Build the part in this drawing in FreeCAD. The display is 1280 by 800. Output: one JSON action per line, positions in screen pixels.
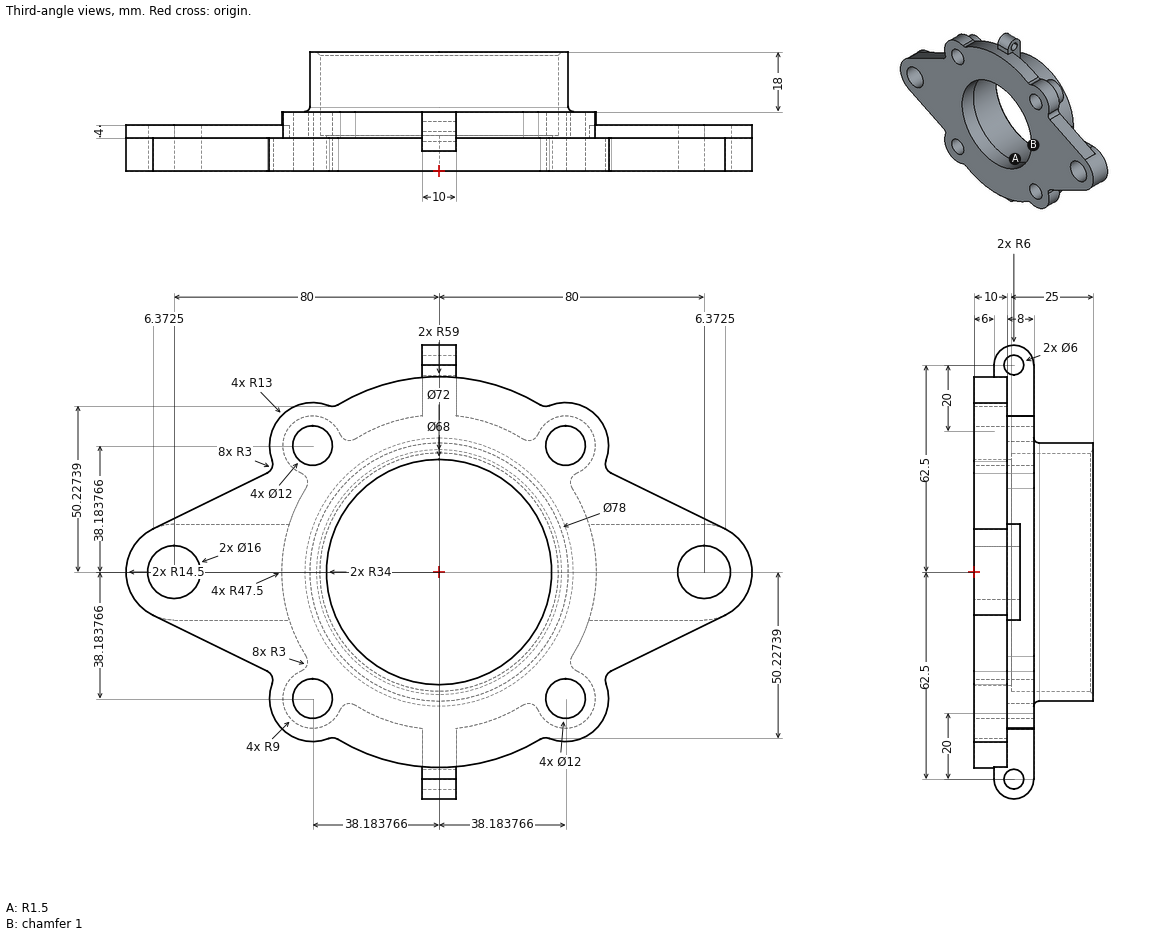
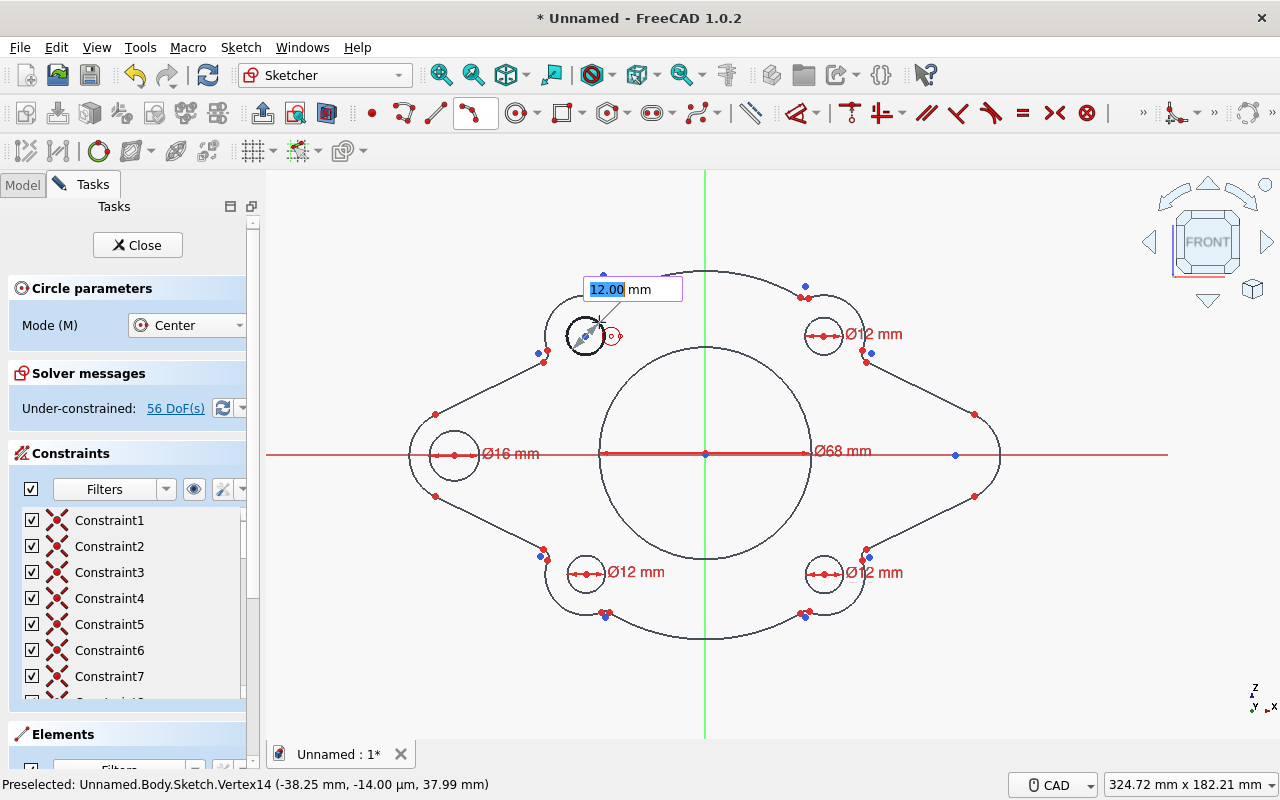
{"action": "type", "text": "12"}
{"action": "key", "text": "Return"}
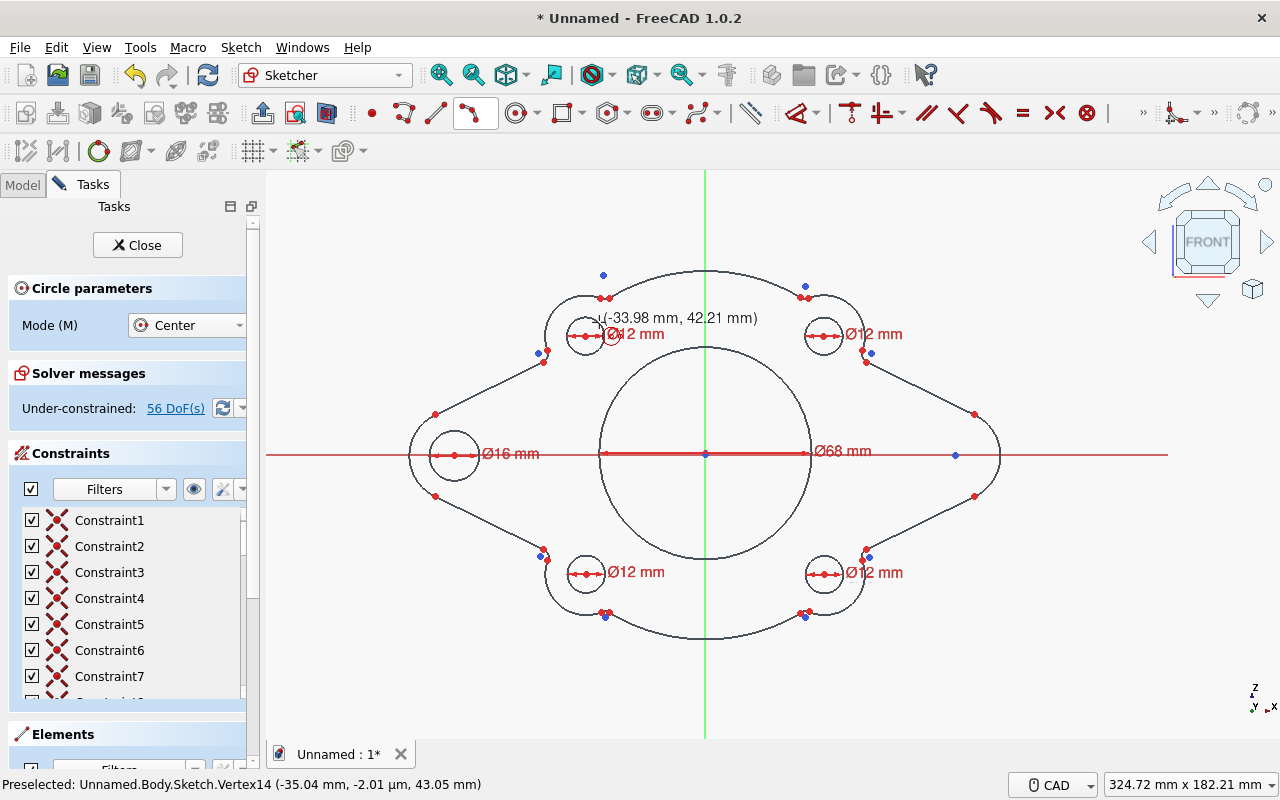
{"action": "left_click", "coordinate": [955, 455]}
{"action": "mouse_move", "coordinate": [973, 437]}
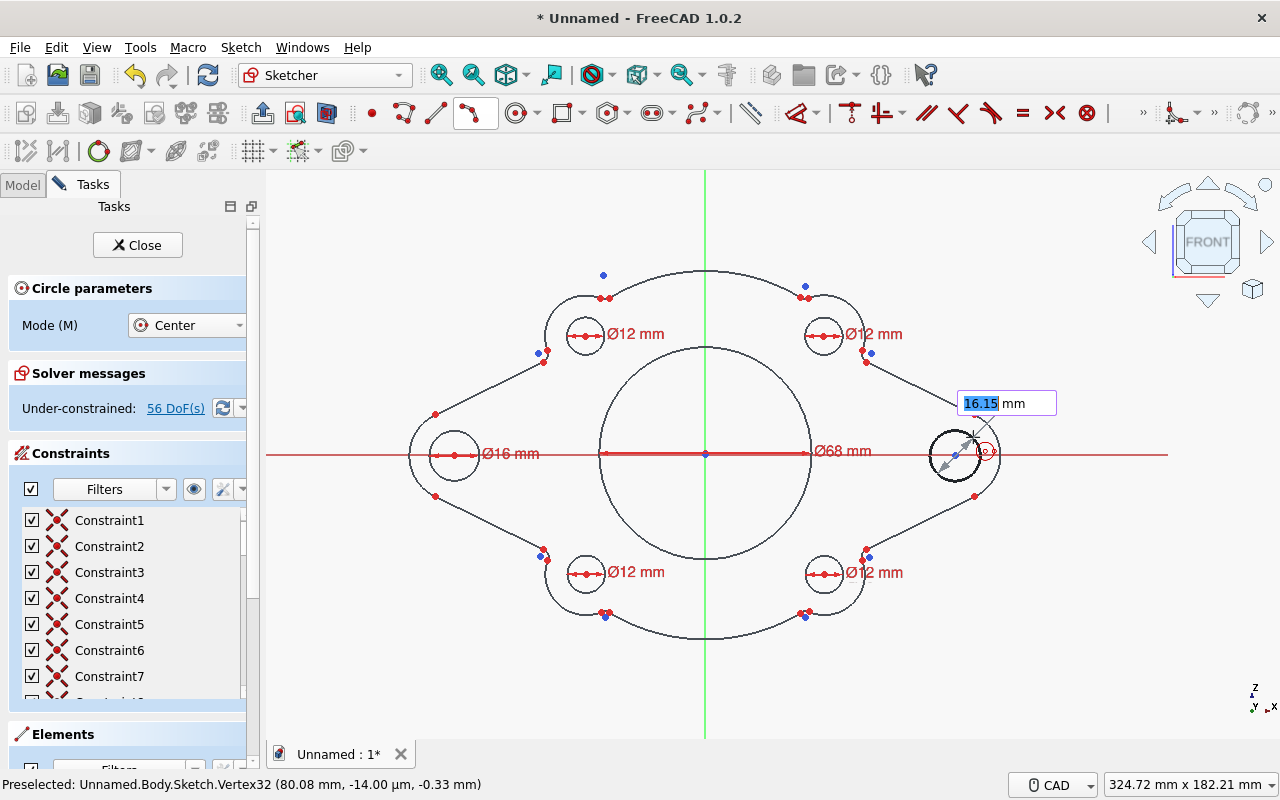
{"action": "type", "text": "16"}
{"action": "key", "text": "Return"}
{"action": "key", "text": "Escape"}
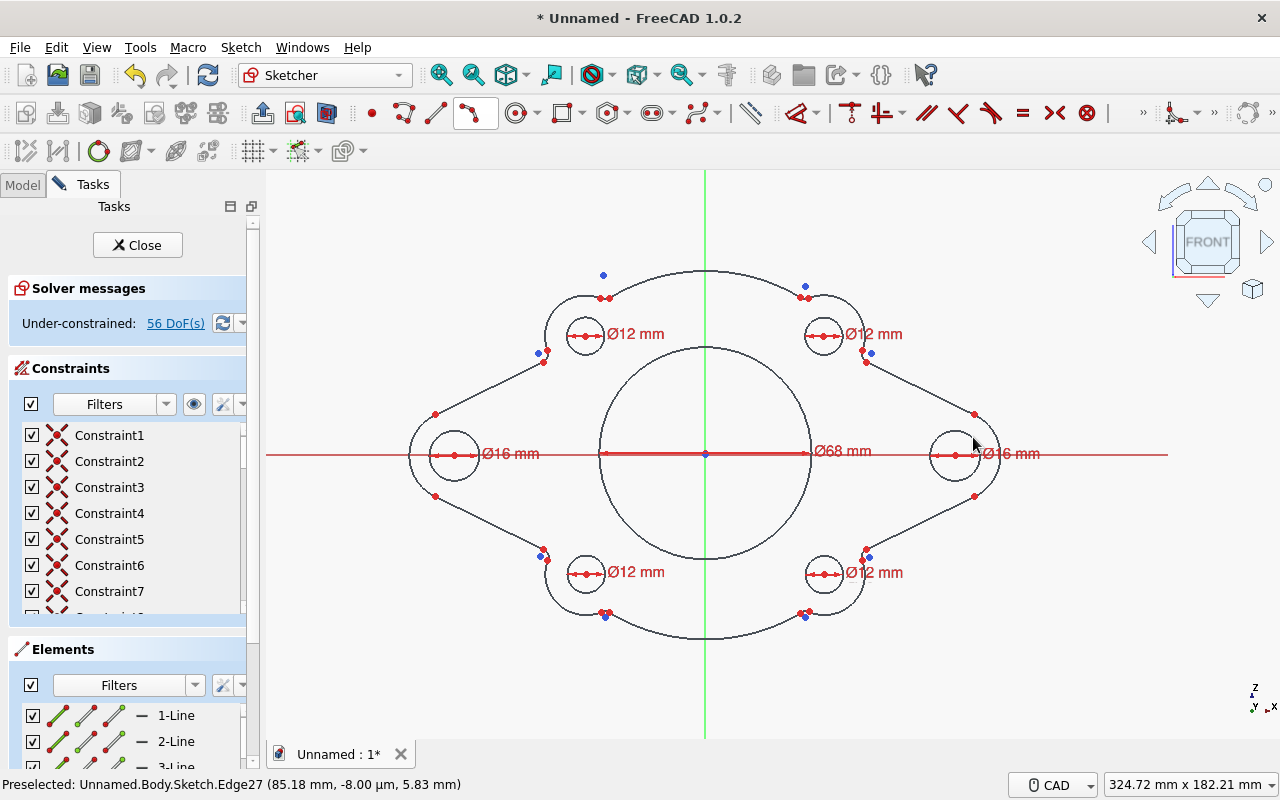
{"action": "left_click", "coordinate": [468, 399]}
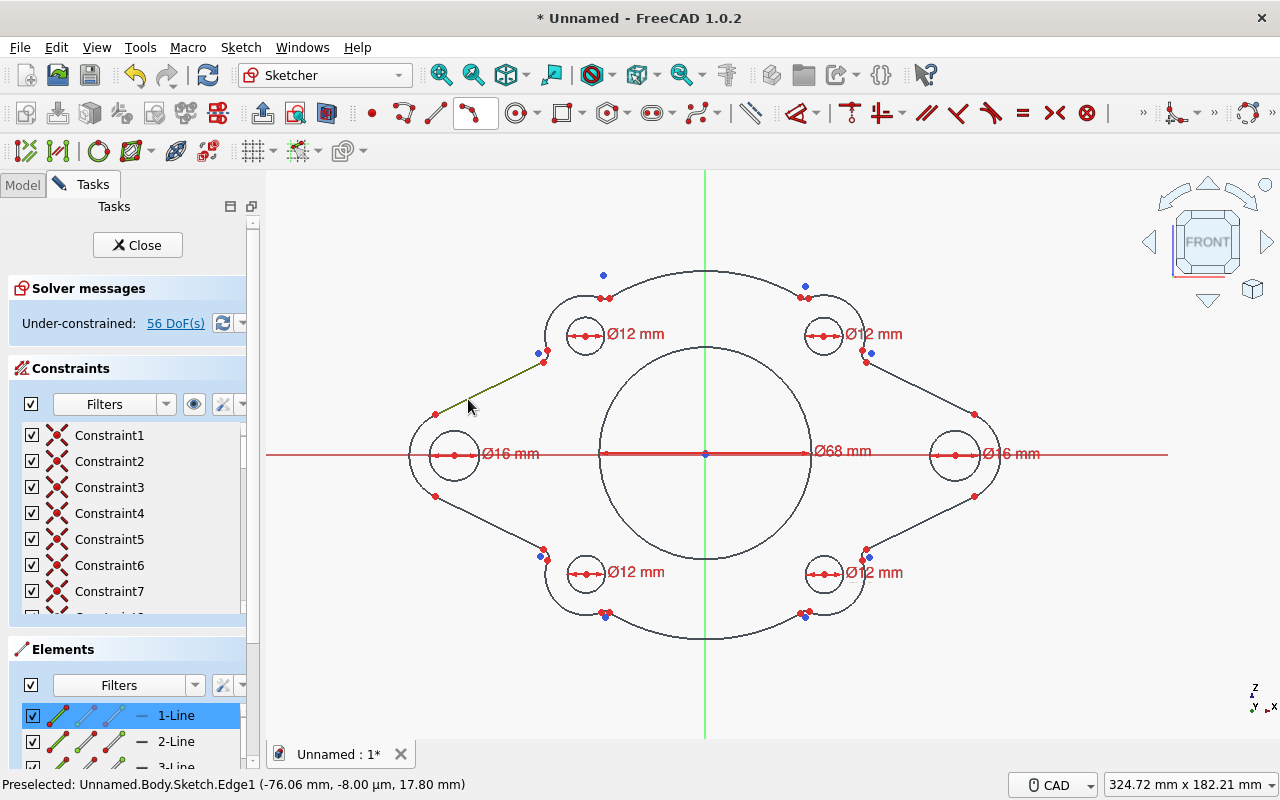
{"action": "scroll", "coordinate": [547, 357], "scroll_direction": "up", "scroll_amount": 4}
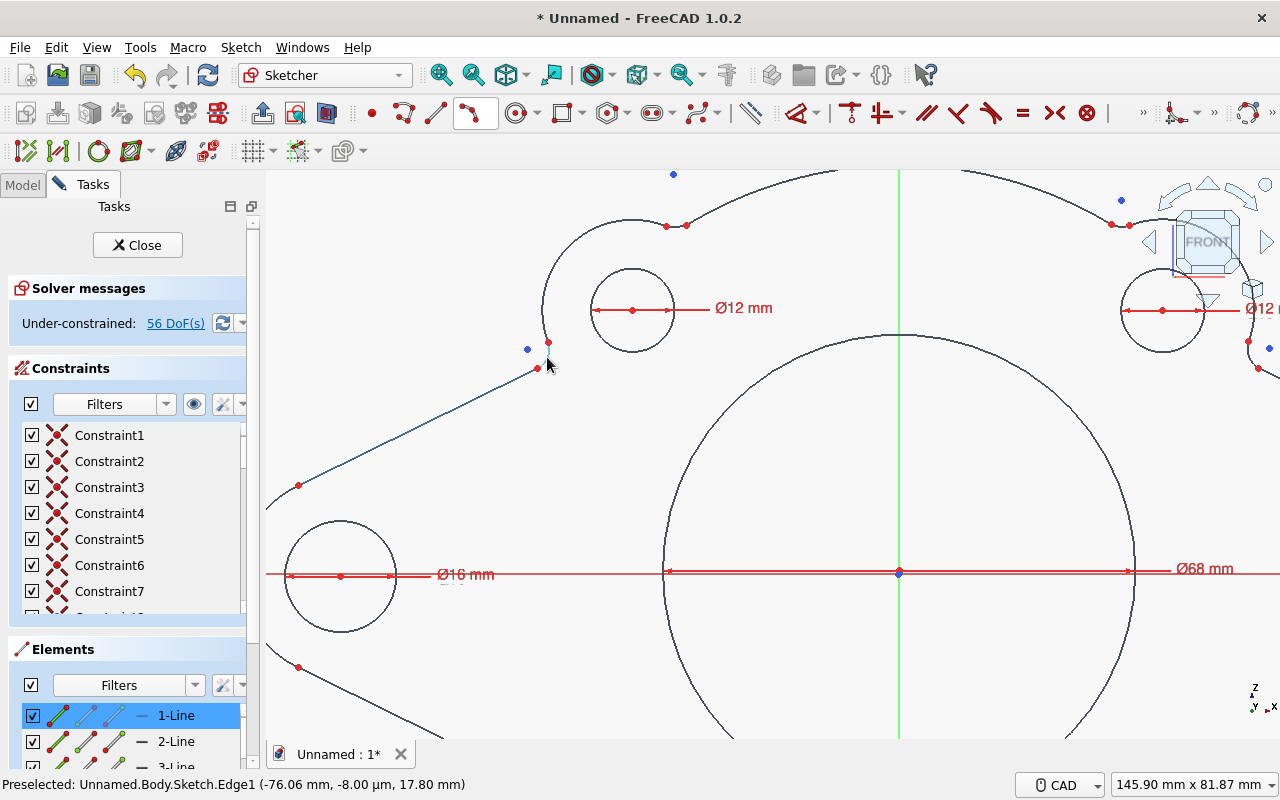
{"action": "left_click", "coordinate": [548, 357]}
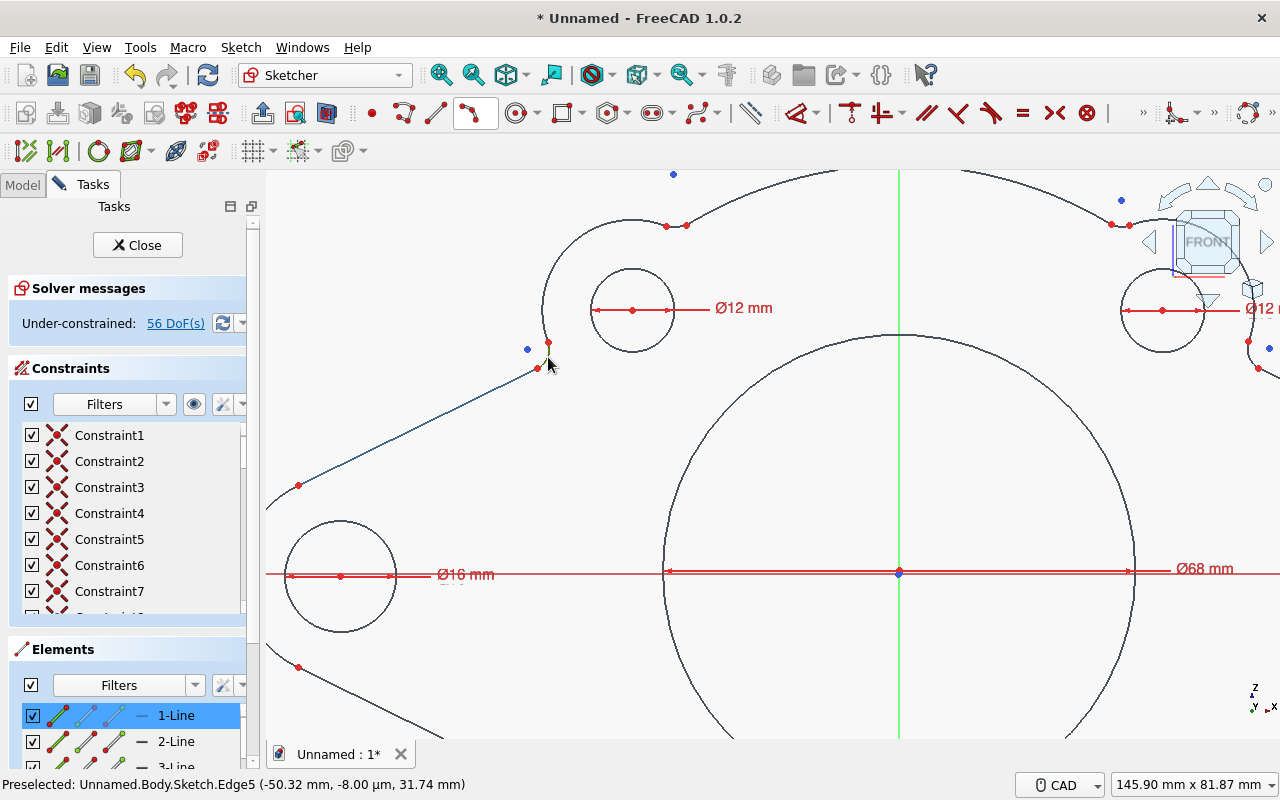
{"action": "left_click", "coordinate": [992, 114]}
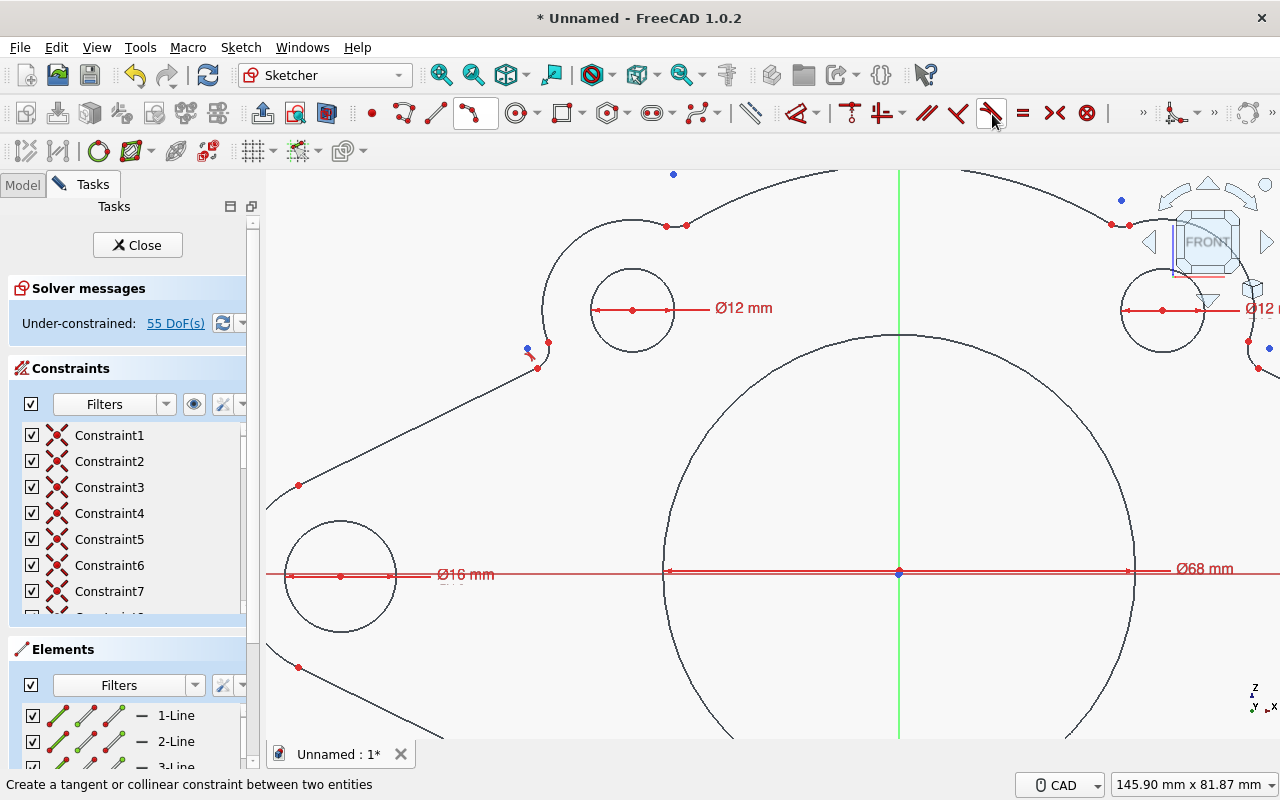
{"action": "left_click", "coordinate": [370, 450]}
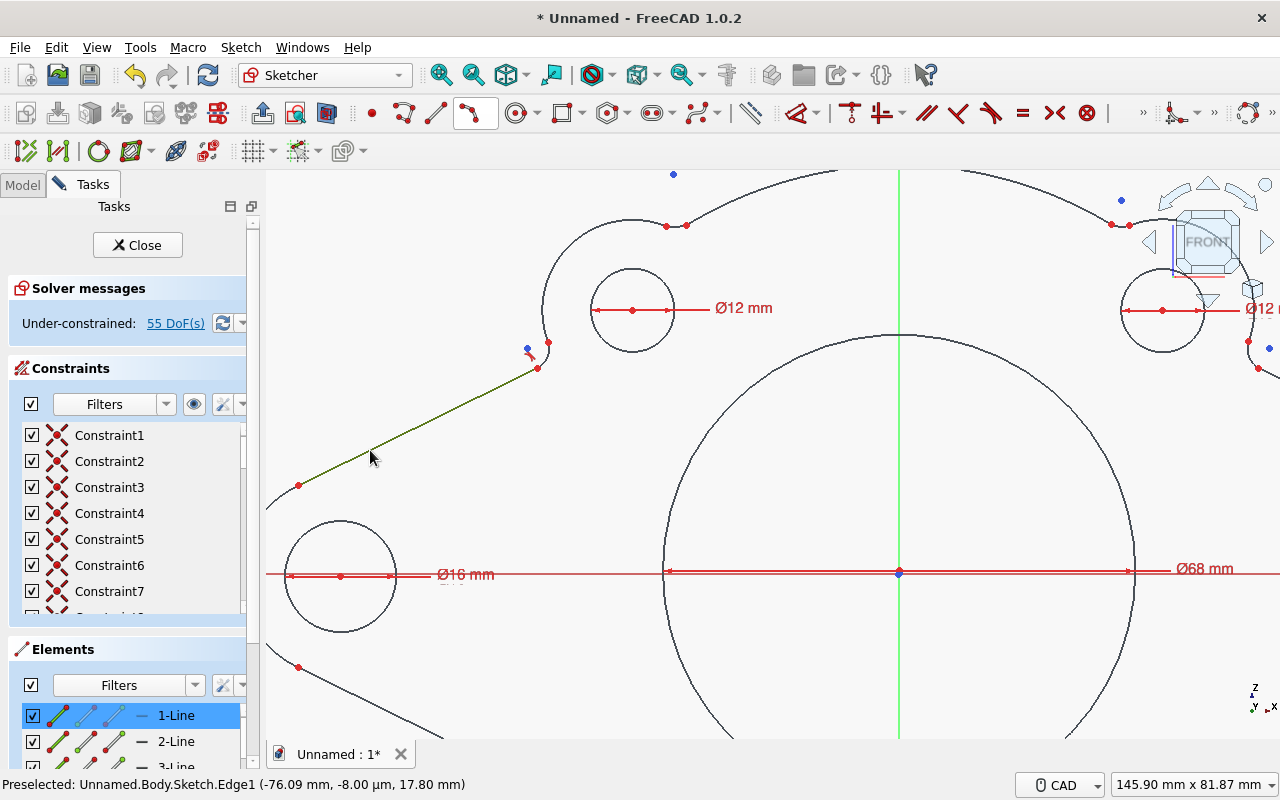
{"action": "scroll", "coordinate": [546, 357], "scroll_direction": "down", "scroll_amount": 4}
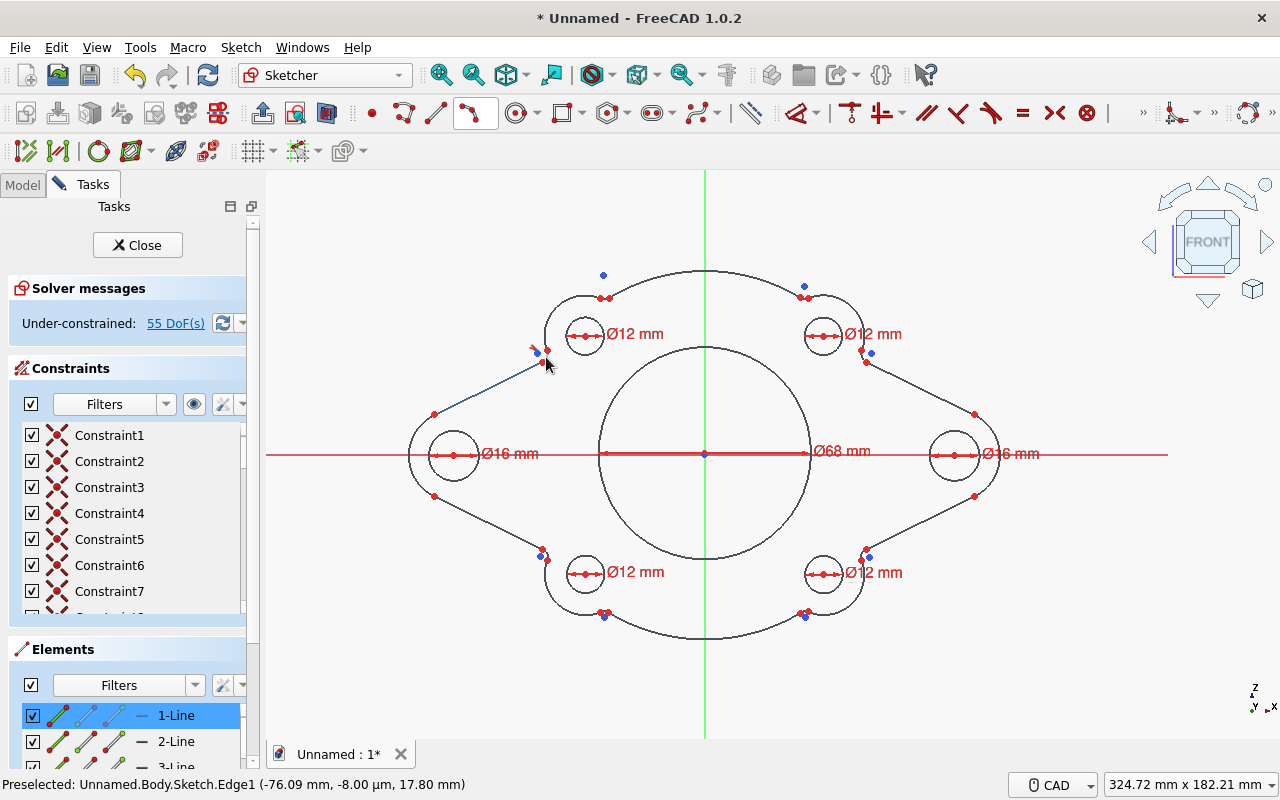
{"action": "left_click", "coordinate": [413, 436]}